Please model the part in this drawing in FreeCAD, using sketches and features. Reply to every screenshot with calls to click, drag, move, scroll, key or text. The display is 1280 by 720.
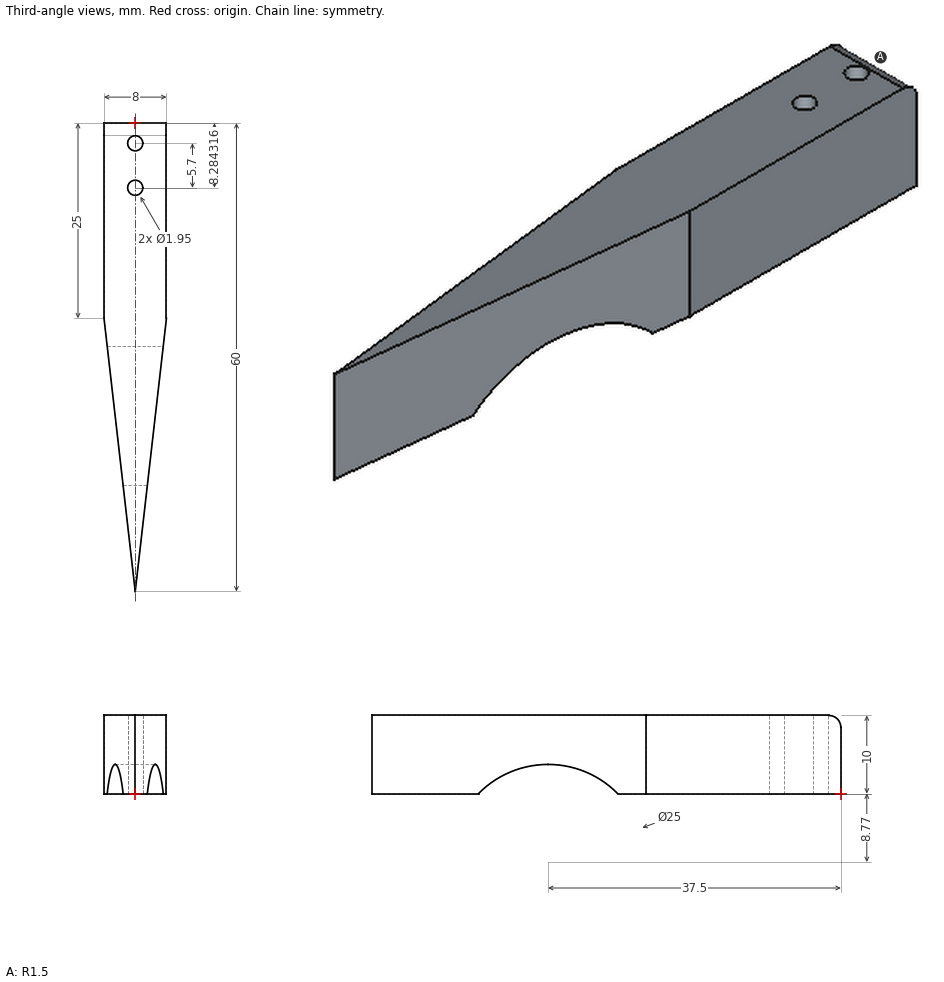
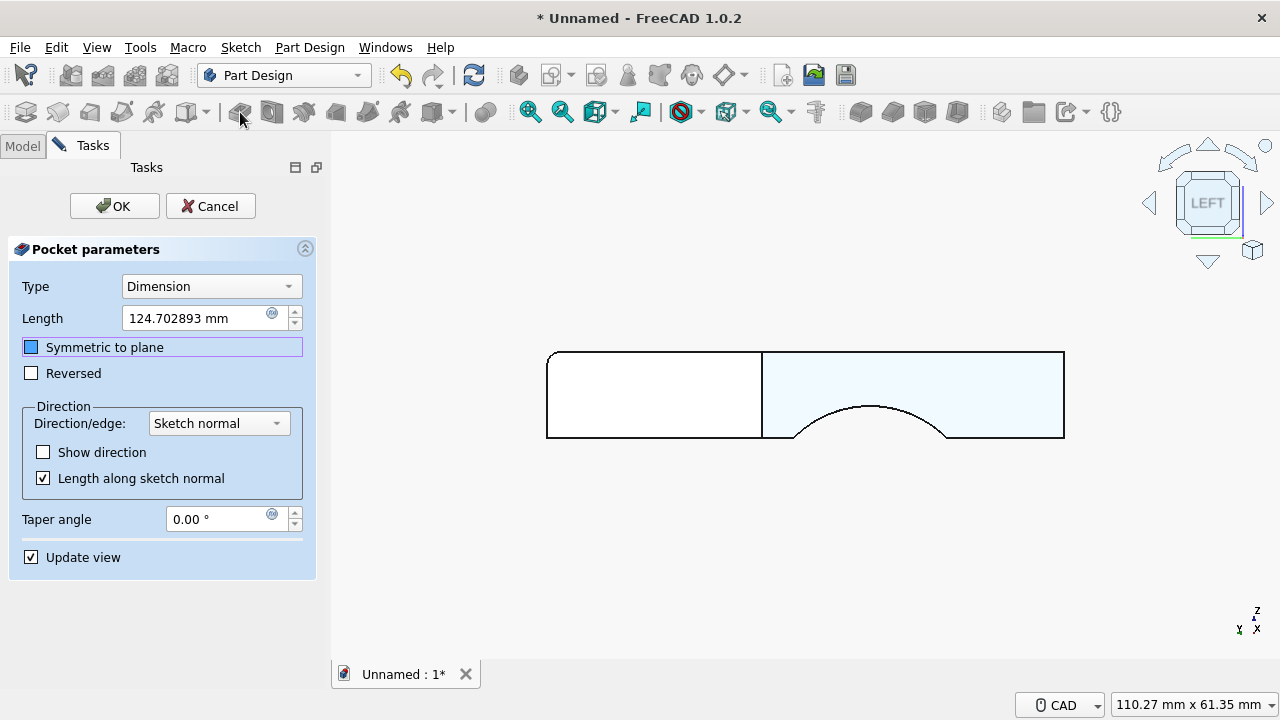
click(30, 347)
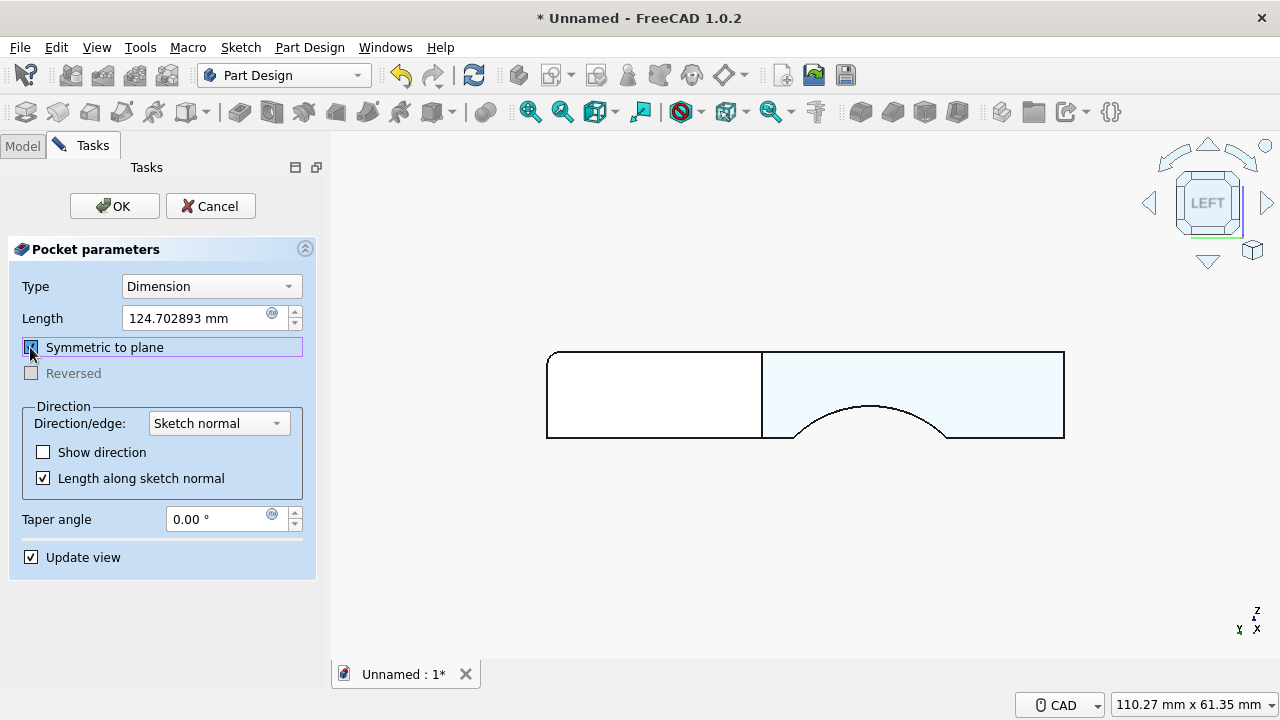
click(115, 206)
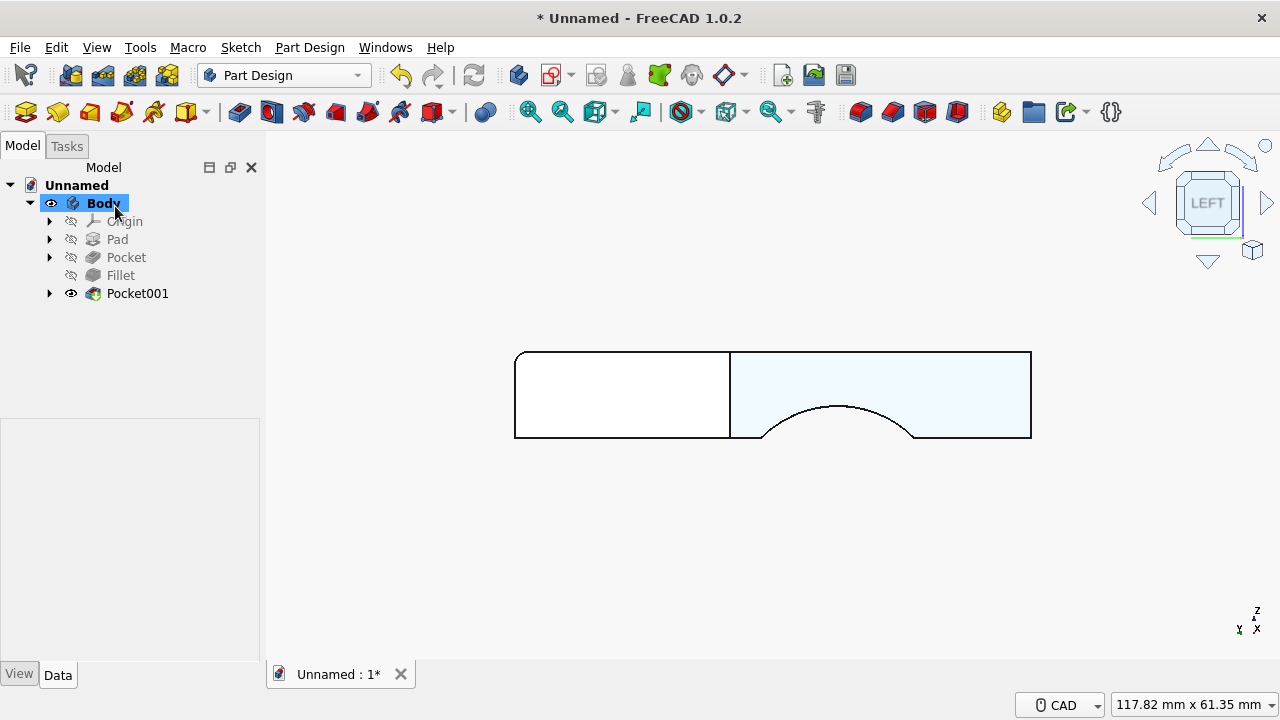
key(0)